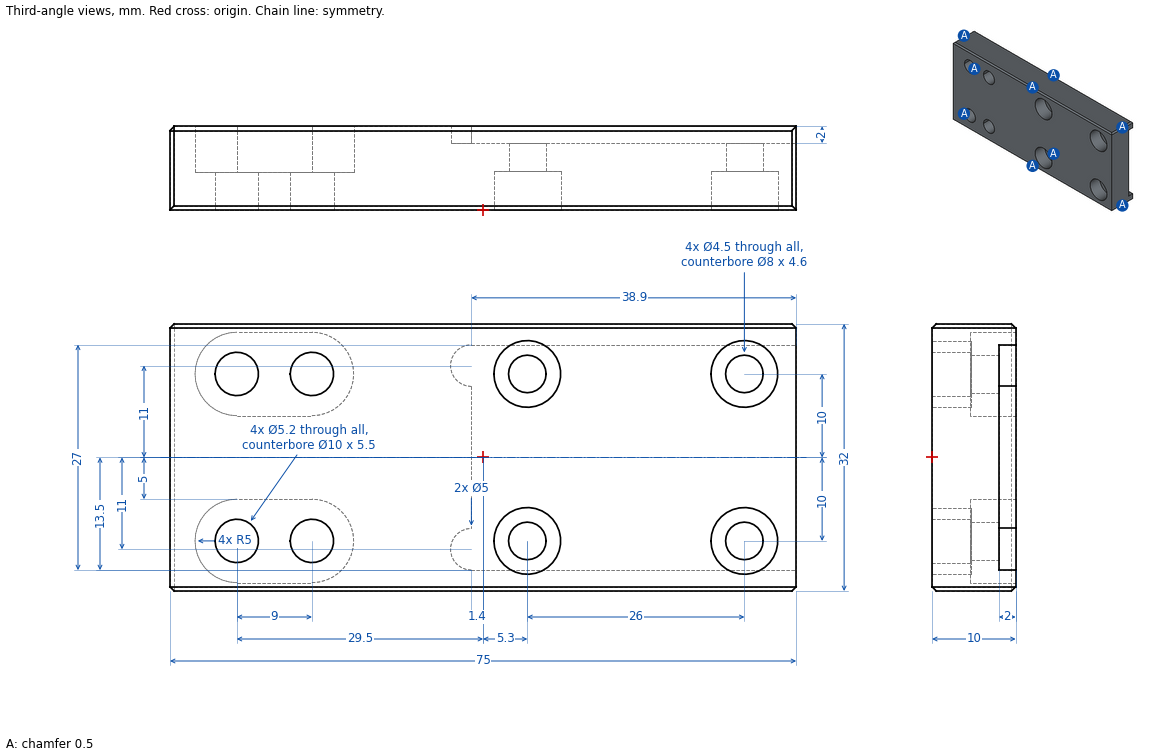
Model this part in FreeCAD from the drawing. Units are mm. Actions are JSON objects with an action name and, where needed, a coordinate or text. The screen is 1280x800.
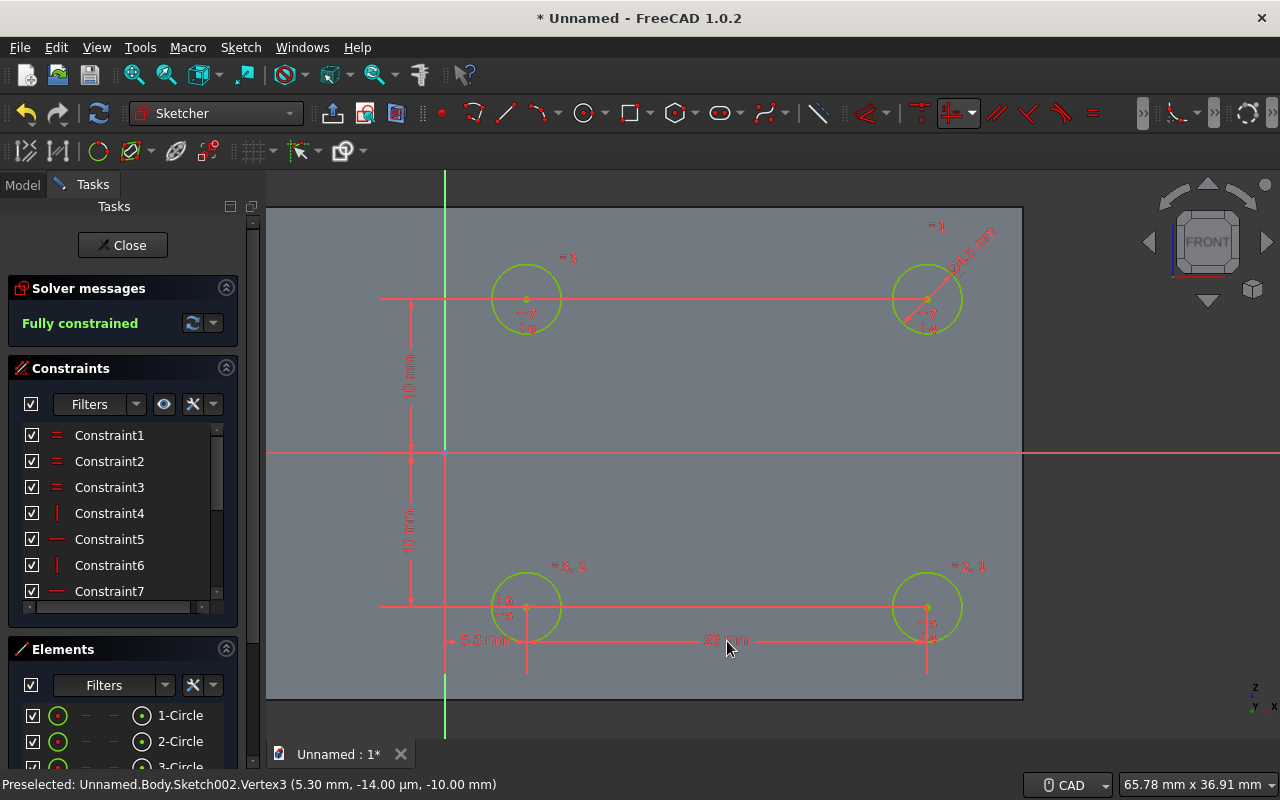
{"action": "left_click", "coordinate": [123, 245]}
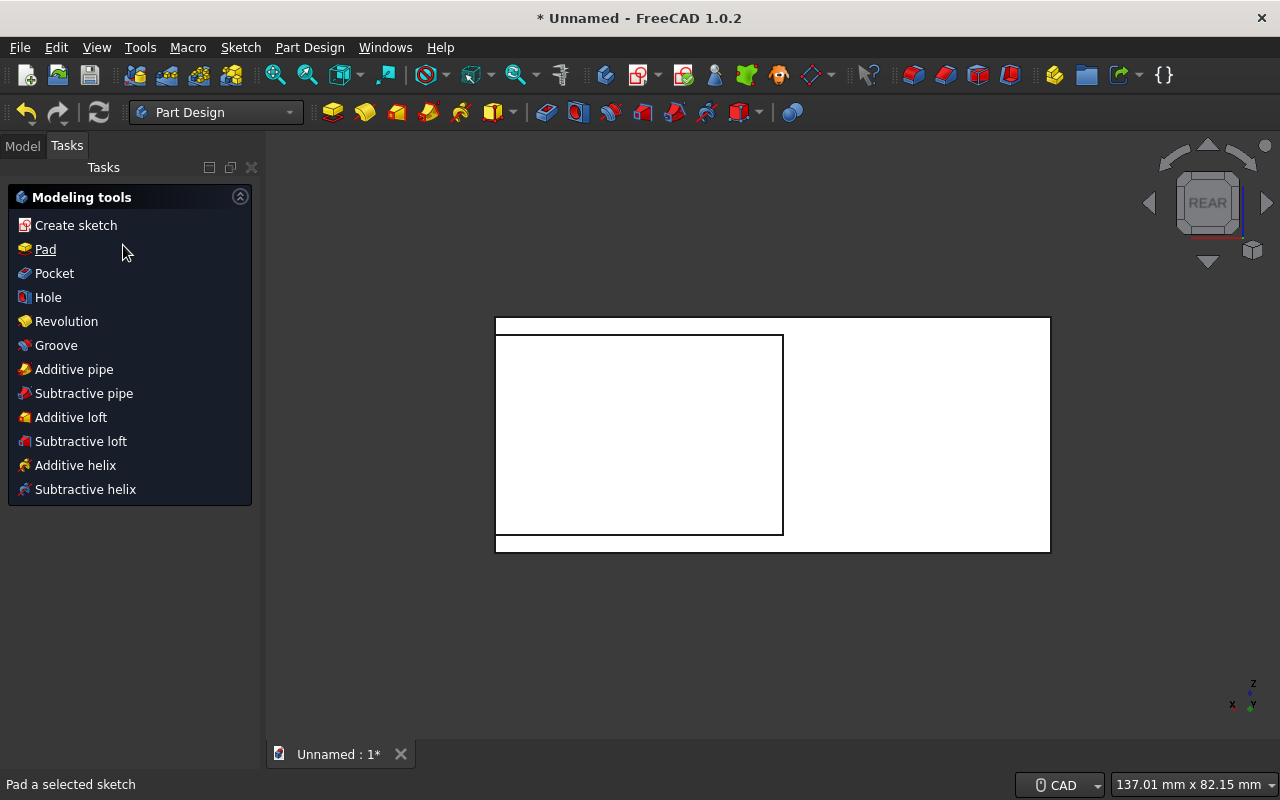
{"action": "left_click", "coordinate": [580, 112]}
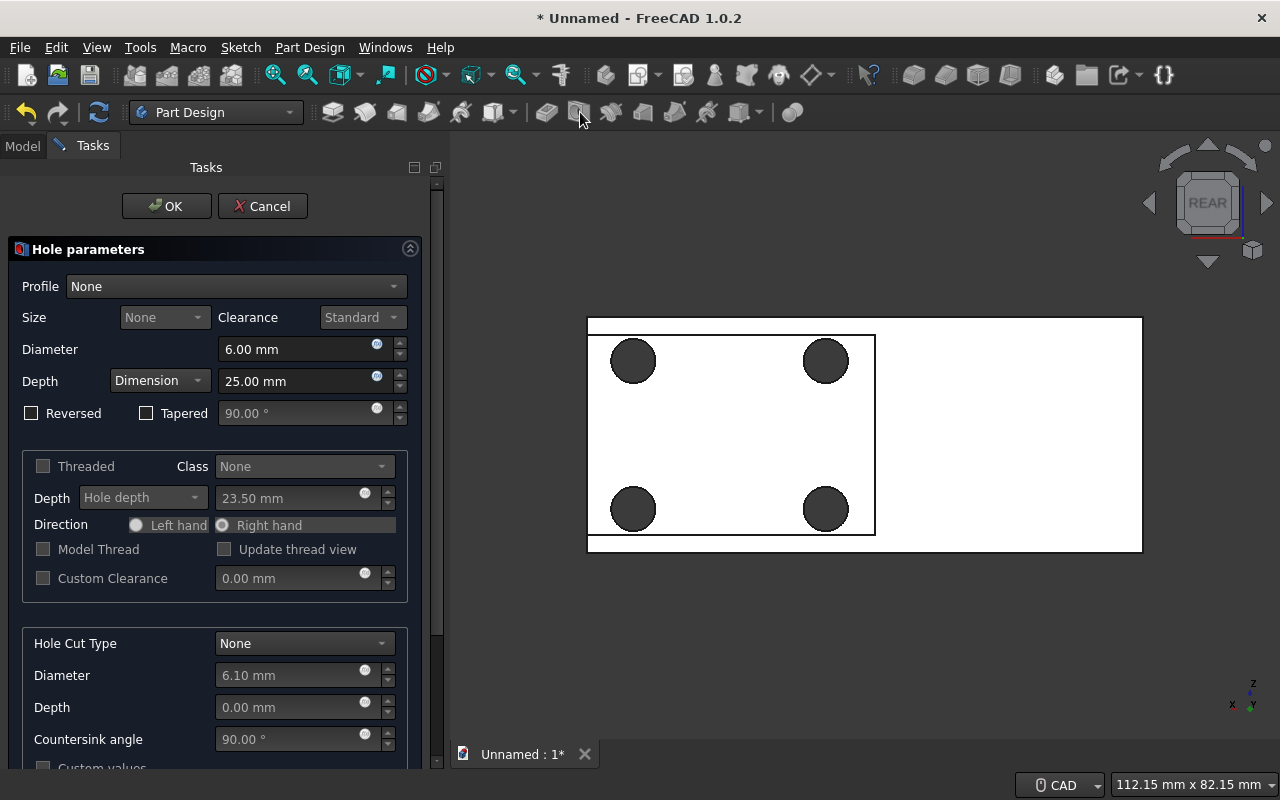
{"action": "triple_click", "coordinate": [305, 349]}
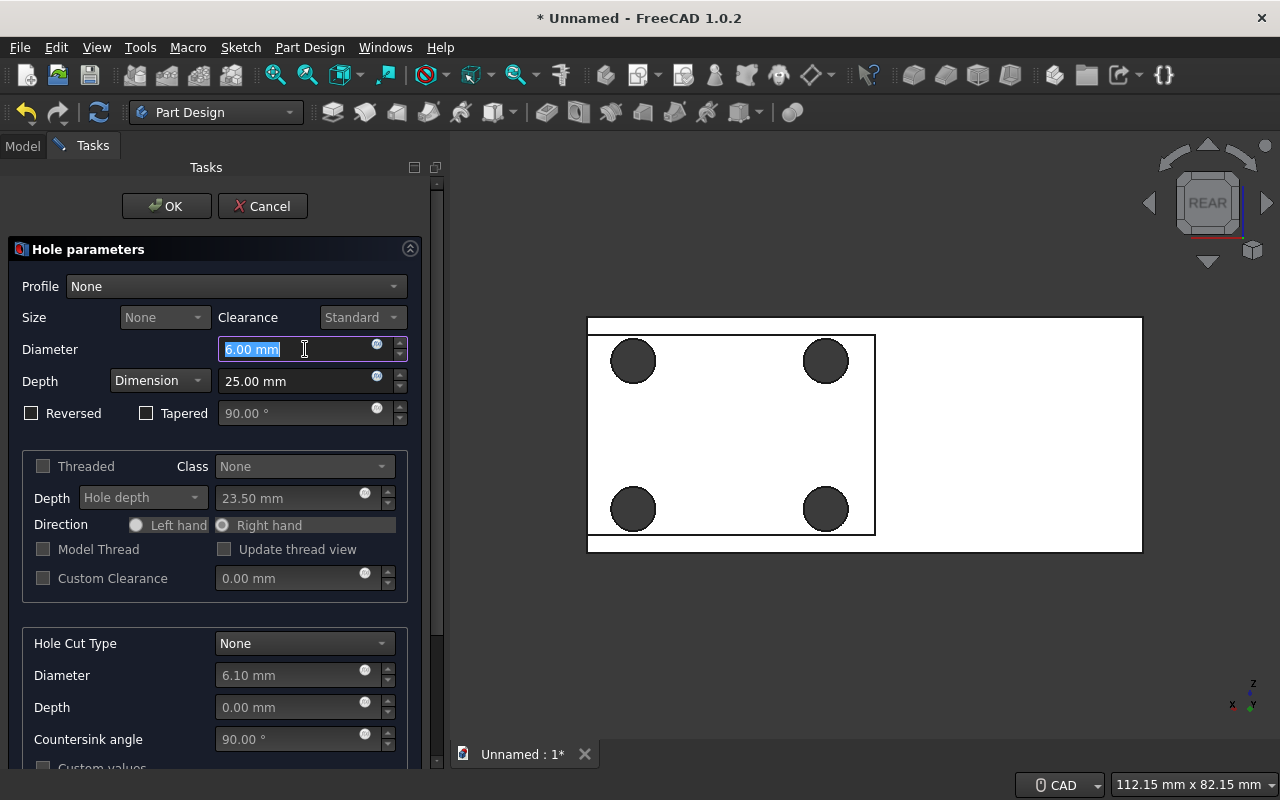
{"action": "type", "text": "4.5"}
{"action": "key", "text": "Tab"}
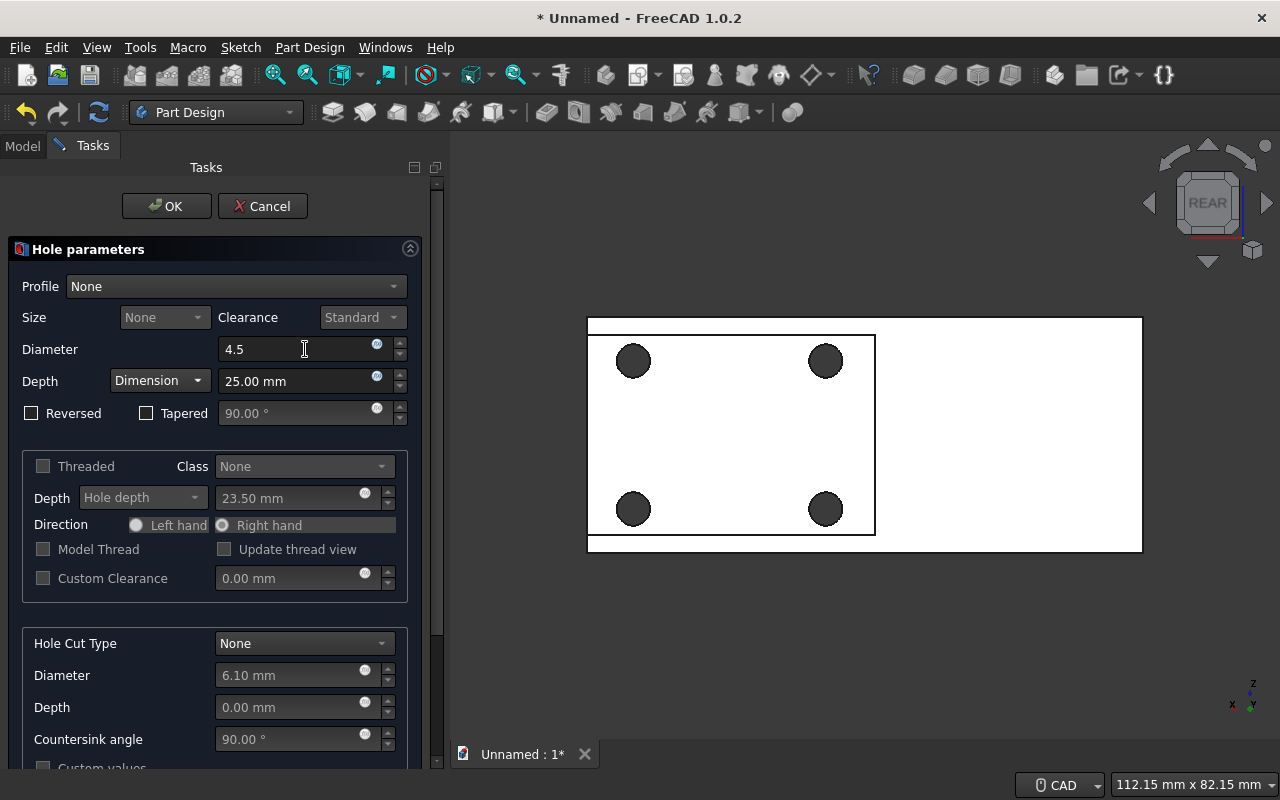
{"action": "left_click", "coordinate": [161, 380]}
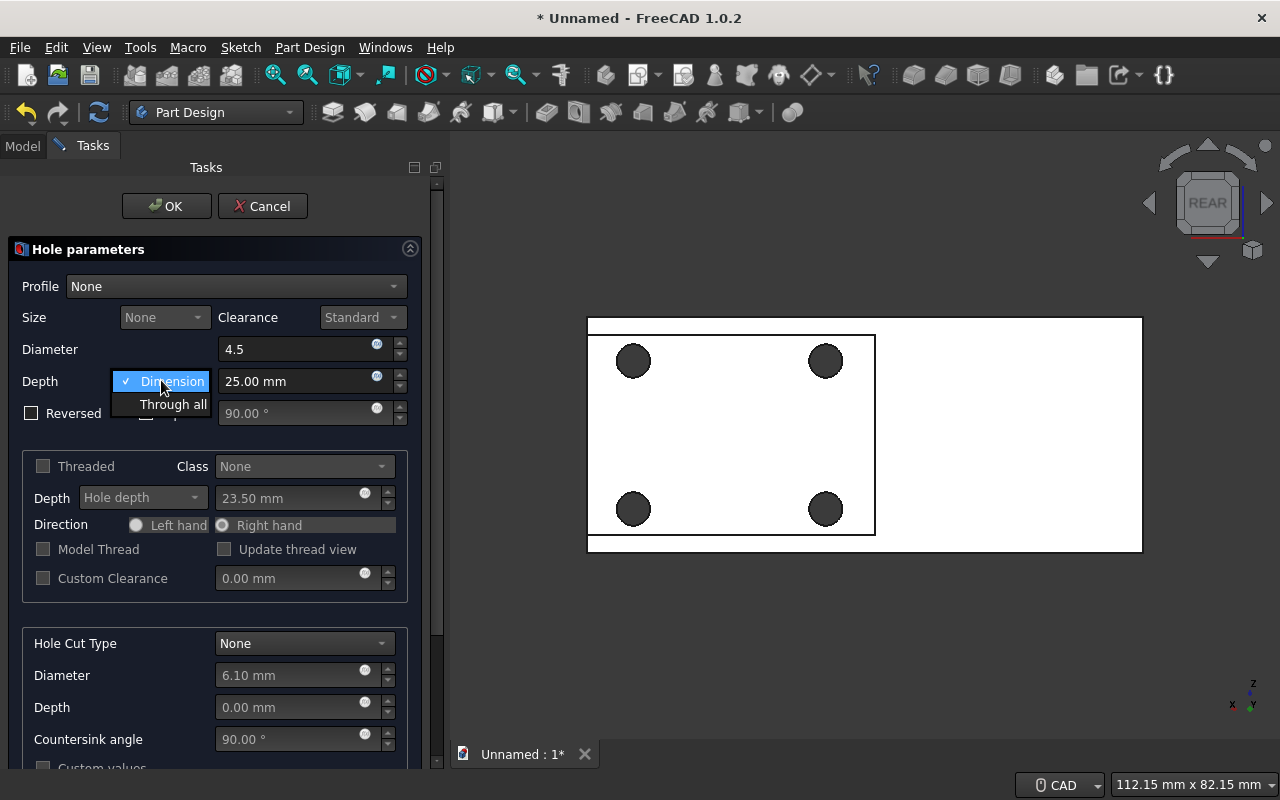
{"action": "left_click", "coordinate": [160, 404]}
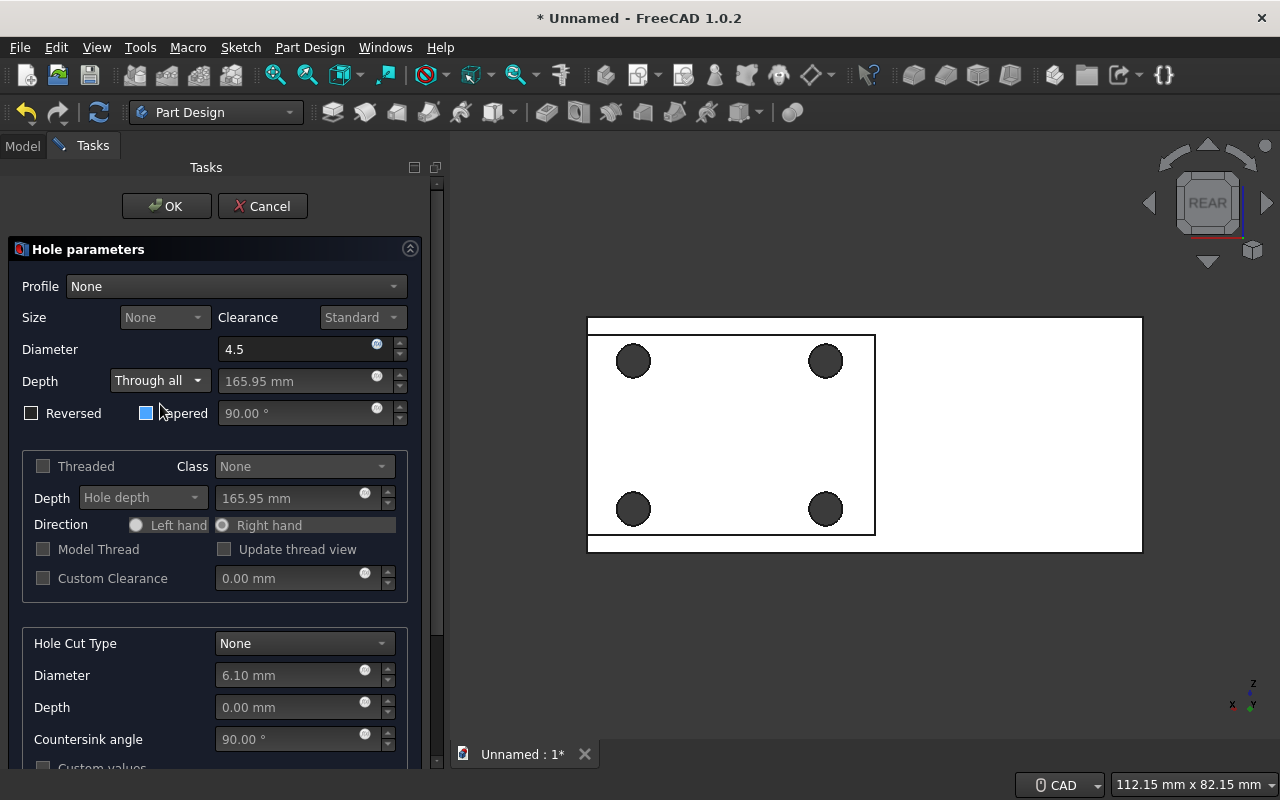
{"action": "left_click", "coordinate": [306, 644]}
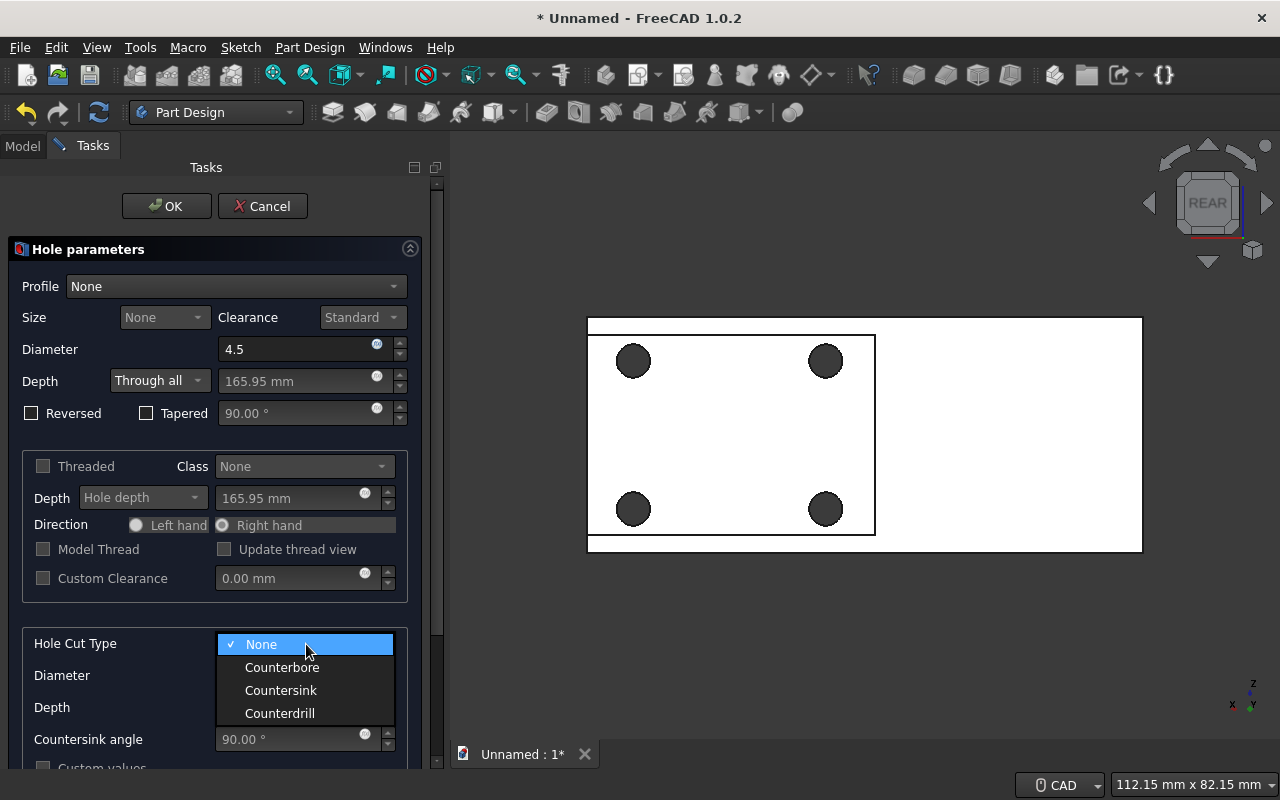
{"action": "left_click", "coordinate": [304, 668]}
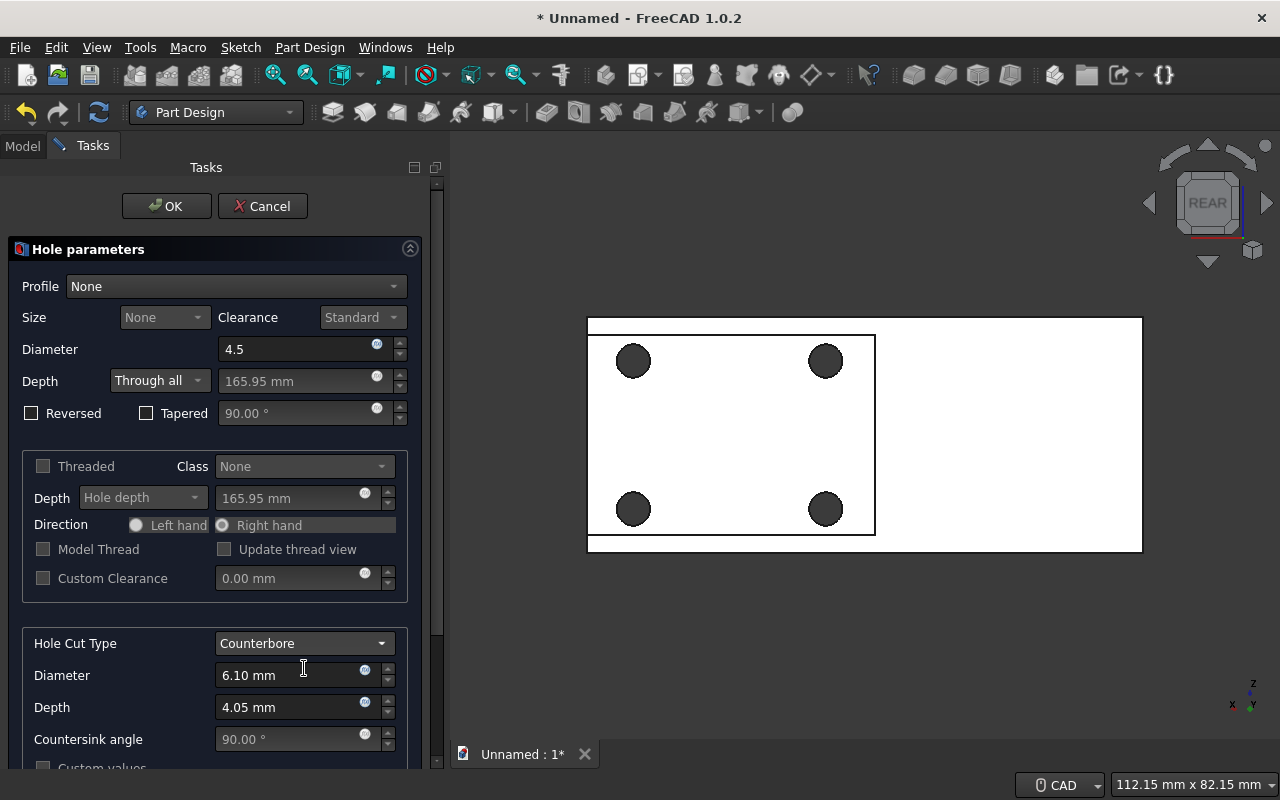
{"action": "triple_click", "coordinate": [298, 675]}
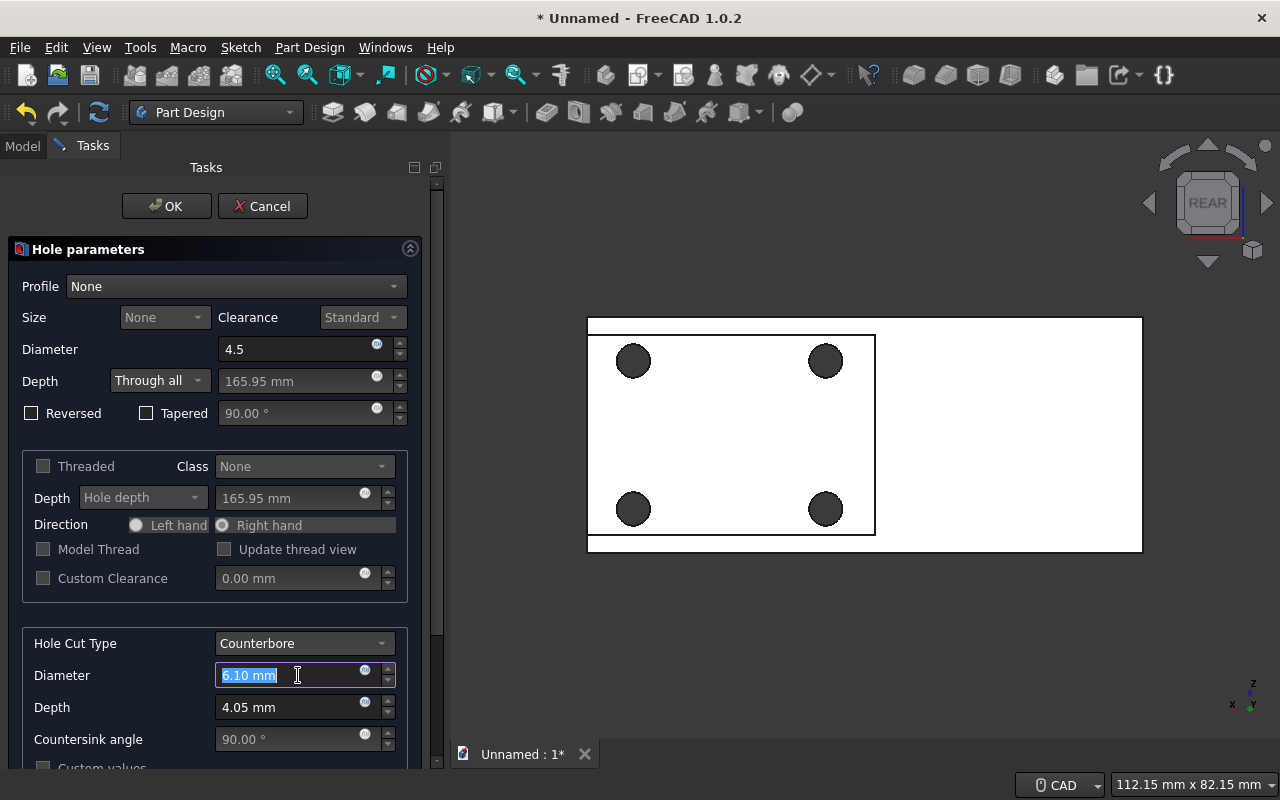
{"action": "type", "text": "8"}
{"action": "key", "text": "Tab"}